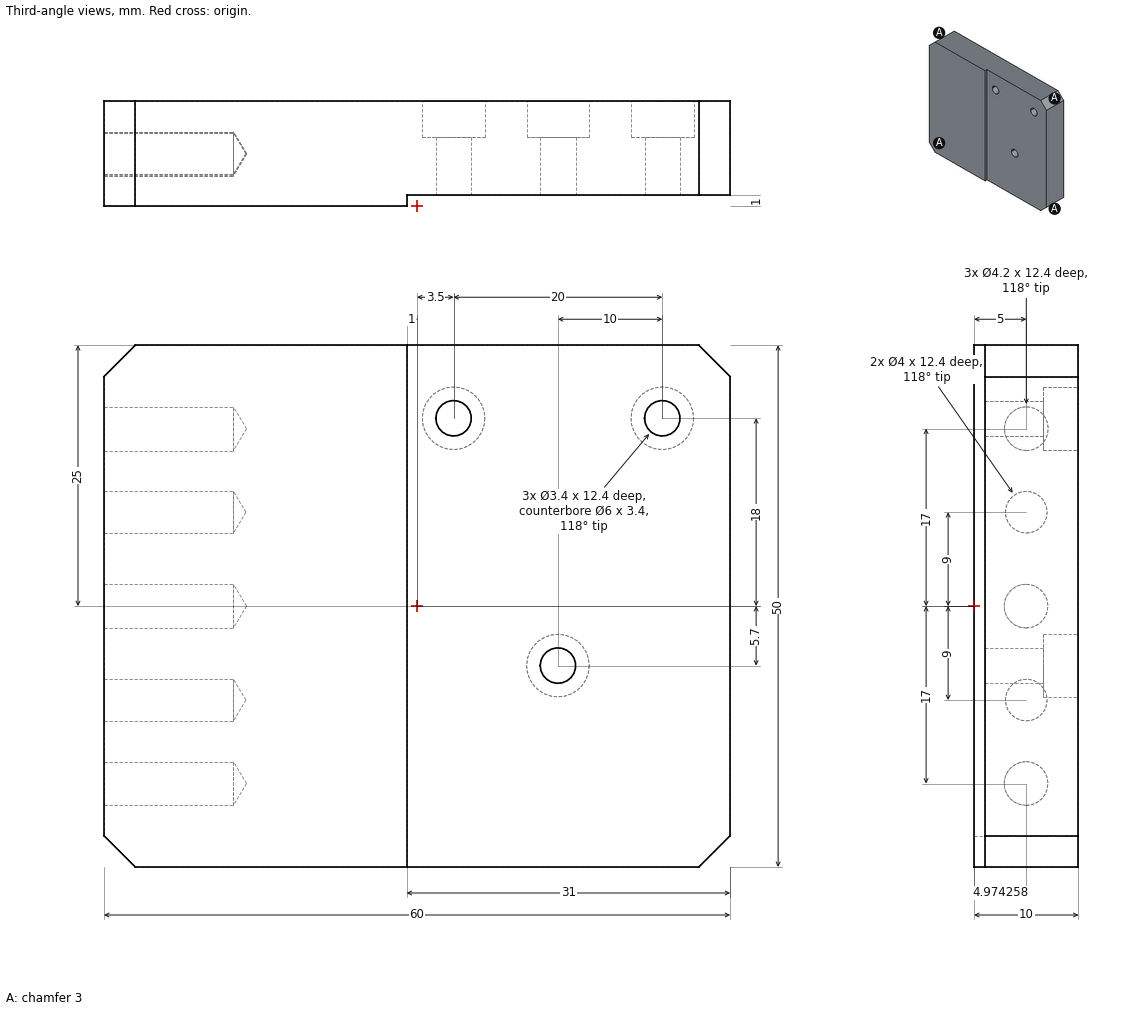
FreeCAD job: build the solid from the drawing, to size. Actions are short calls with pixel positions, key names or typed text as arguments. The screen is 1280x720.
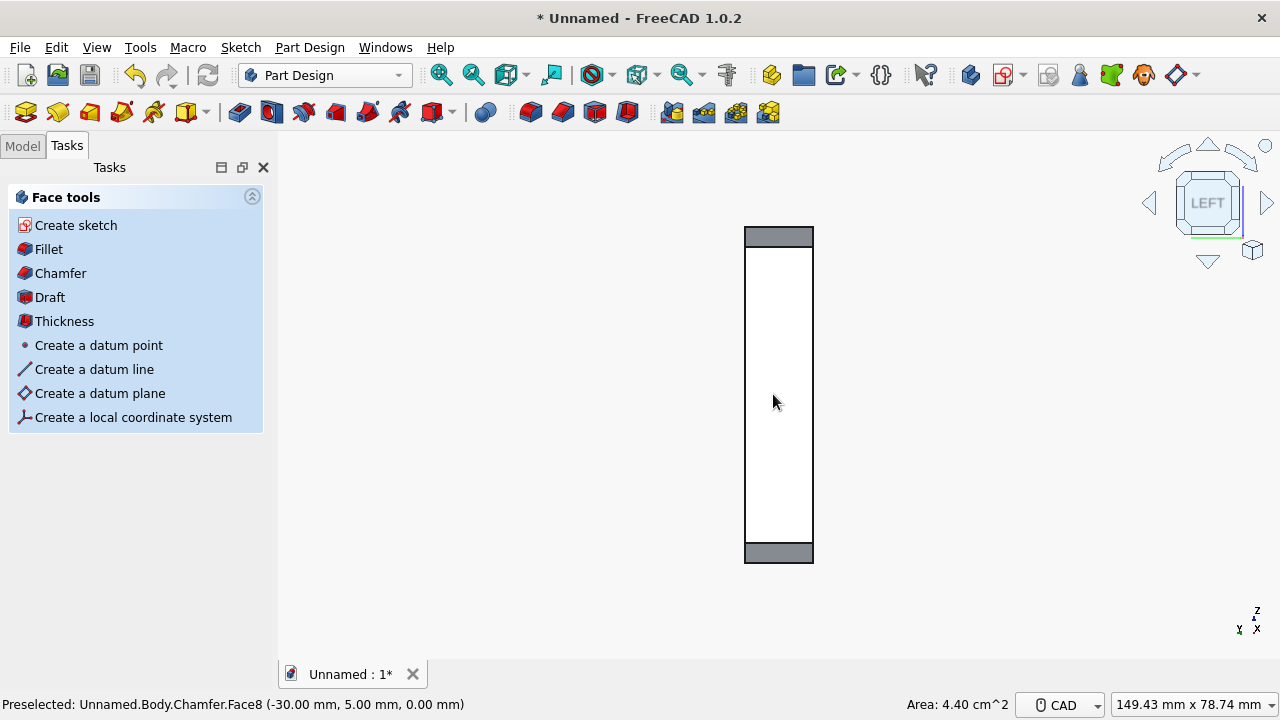
click(1004, 76)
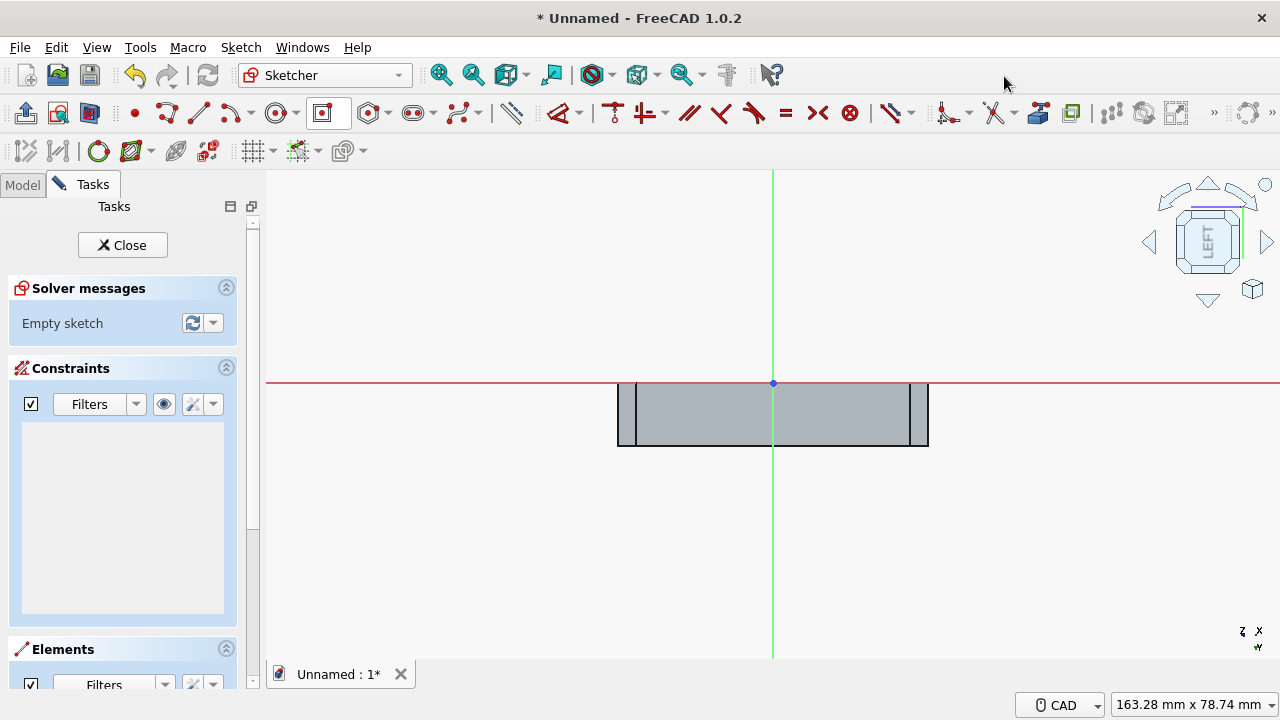
scroll(829, 398, up, 4)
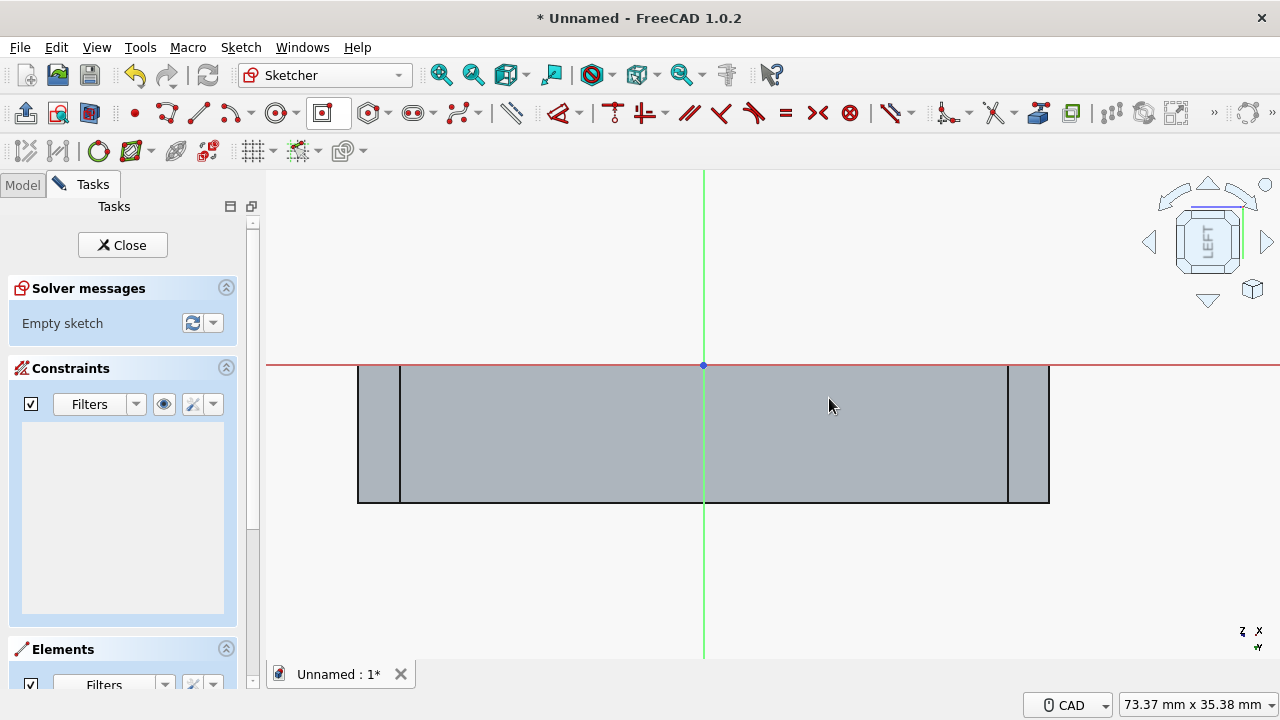
click(276, 114)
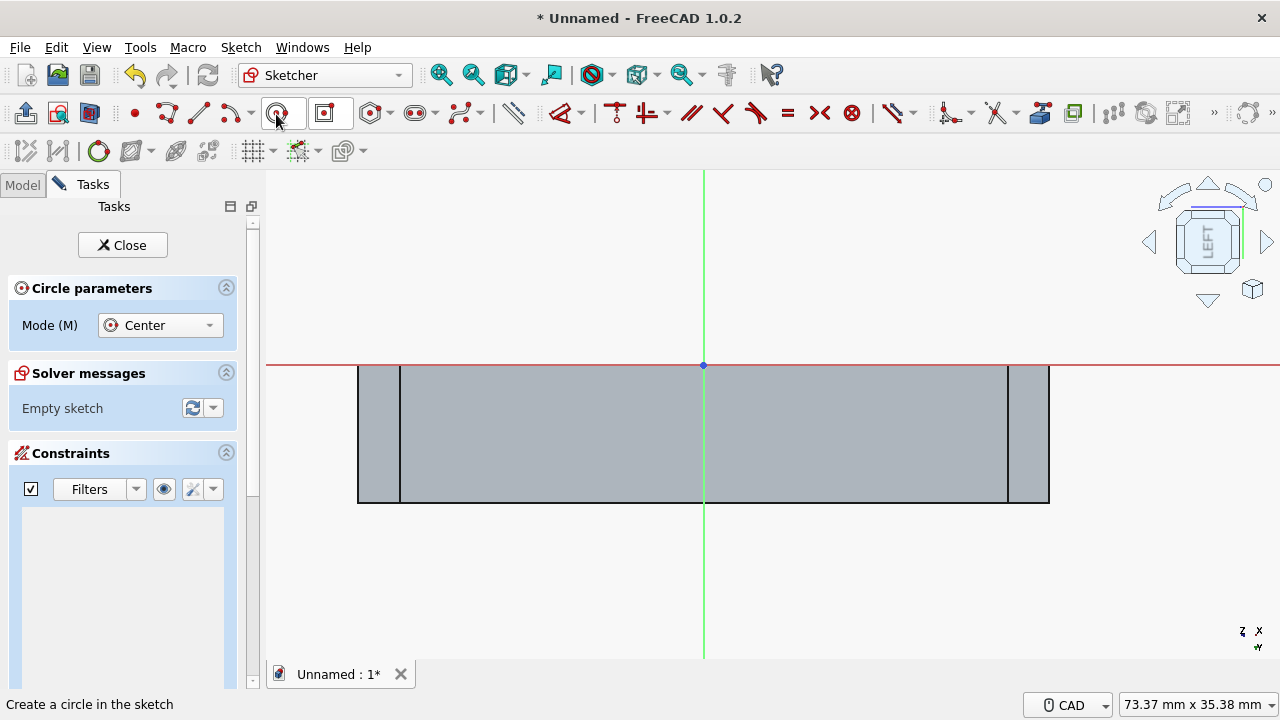
click(469, 434)
move(489, 414)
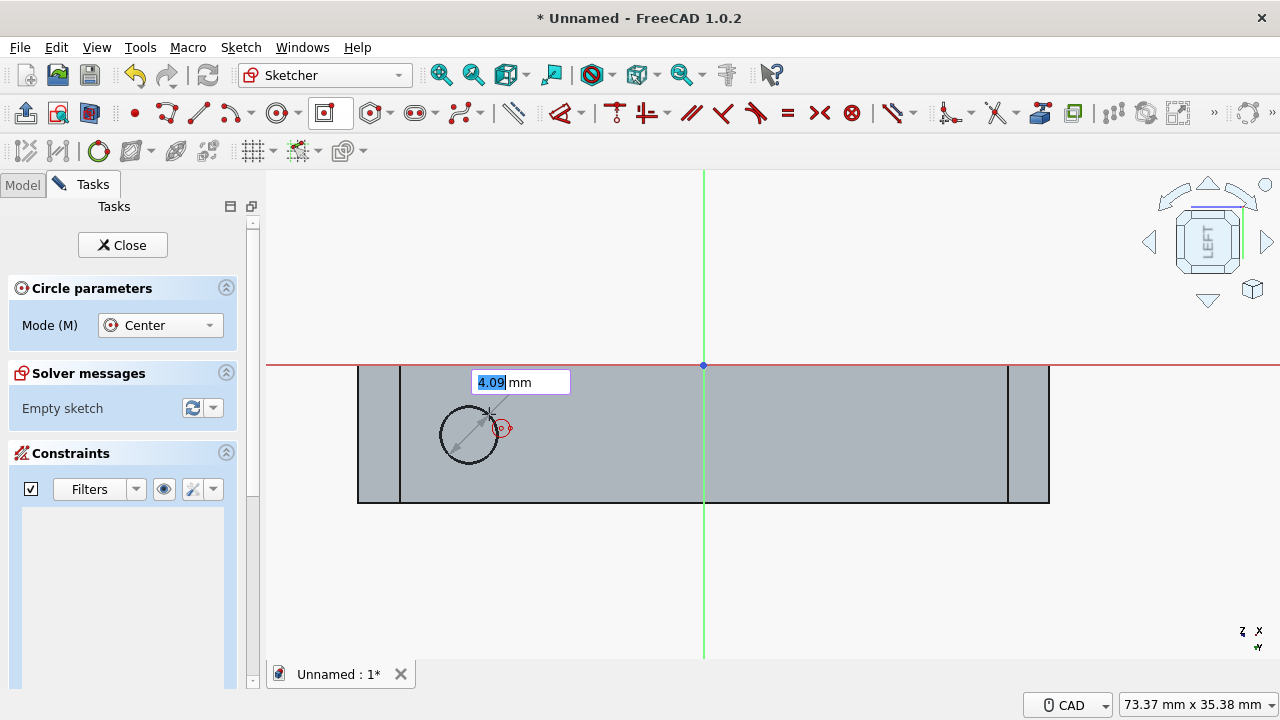
text(4.2)
key(Return)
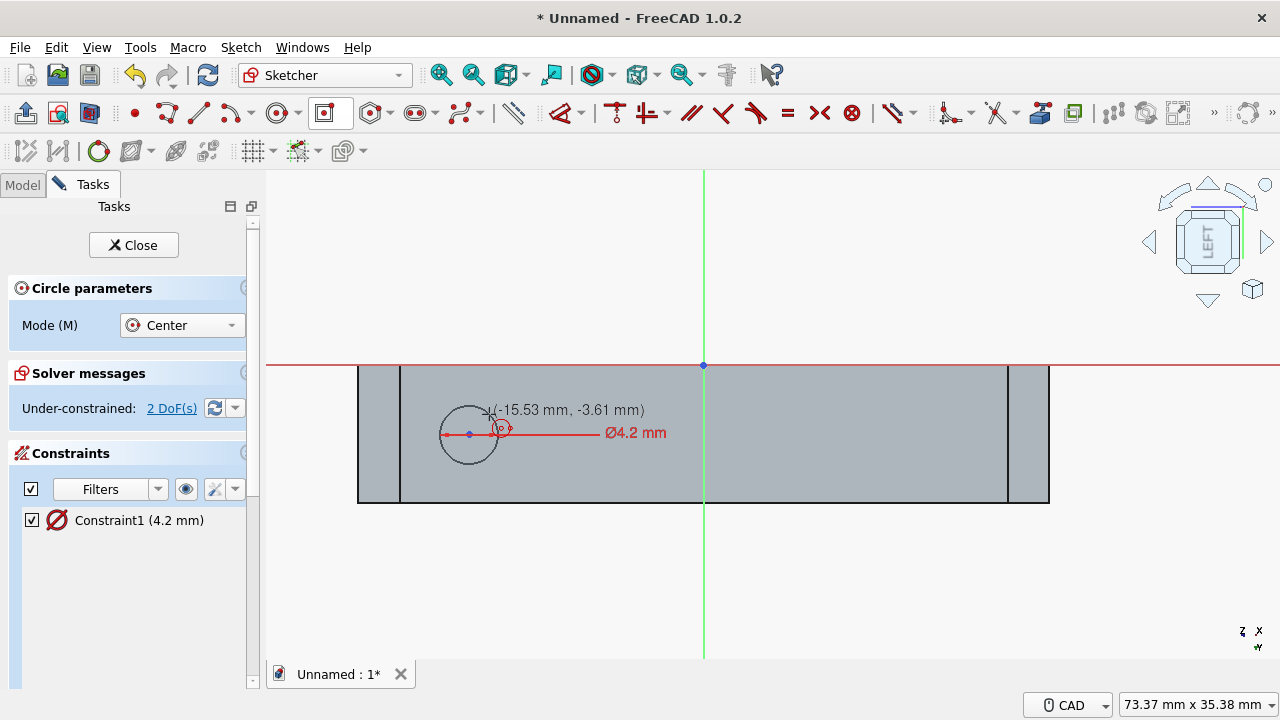
click(939, 434)
move(959, 413)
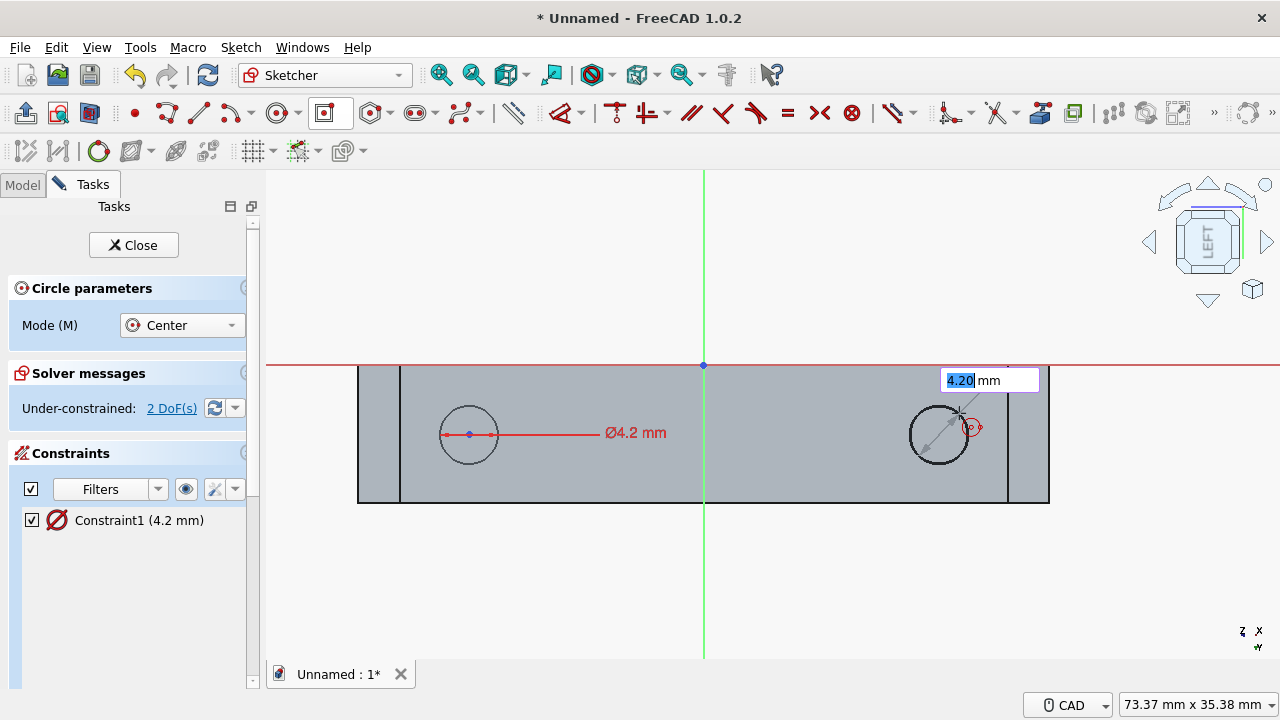
text(4.2)
key(Return)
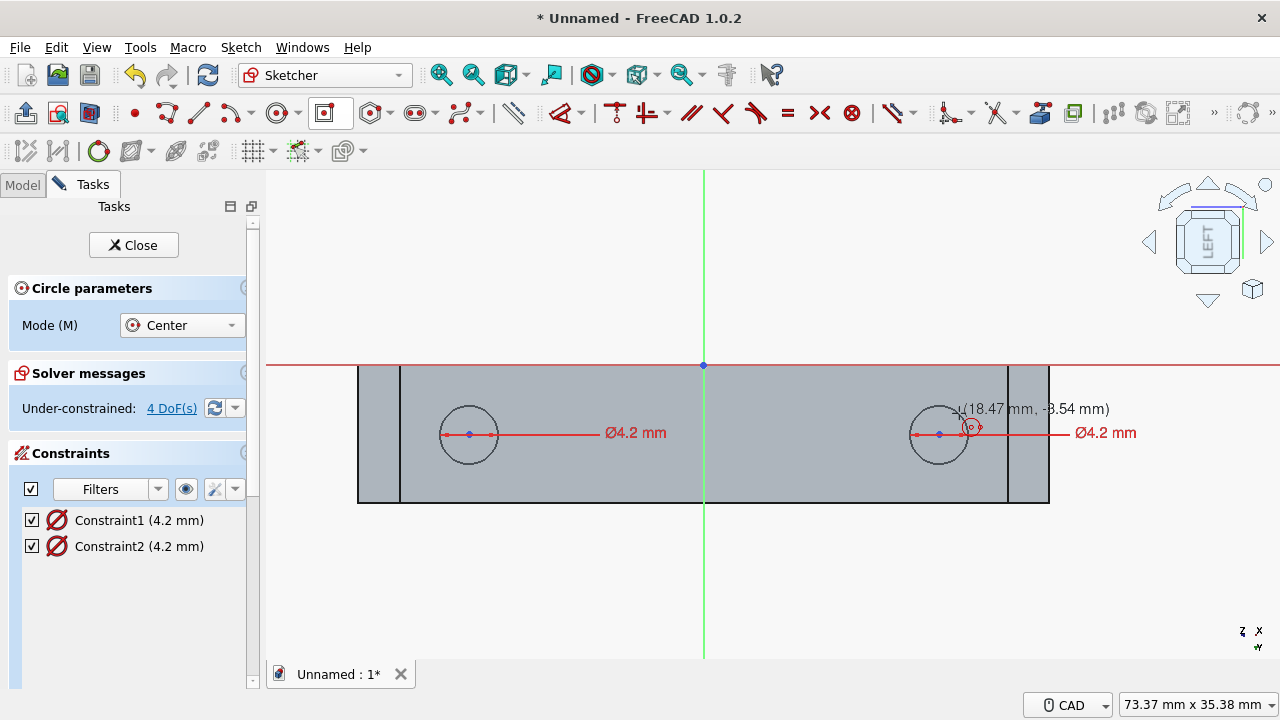
click(704, 434)
move(724, 413)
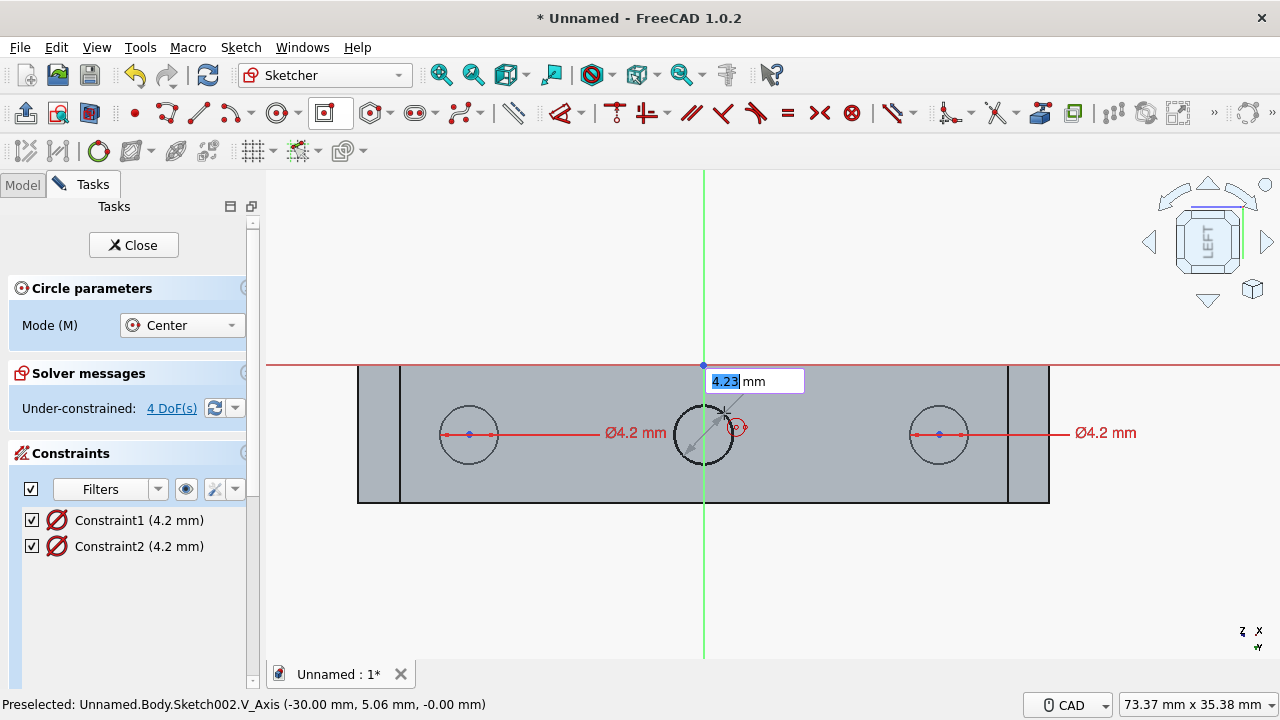
text(4.2)
key(Return)
key(Escape)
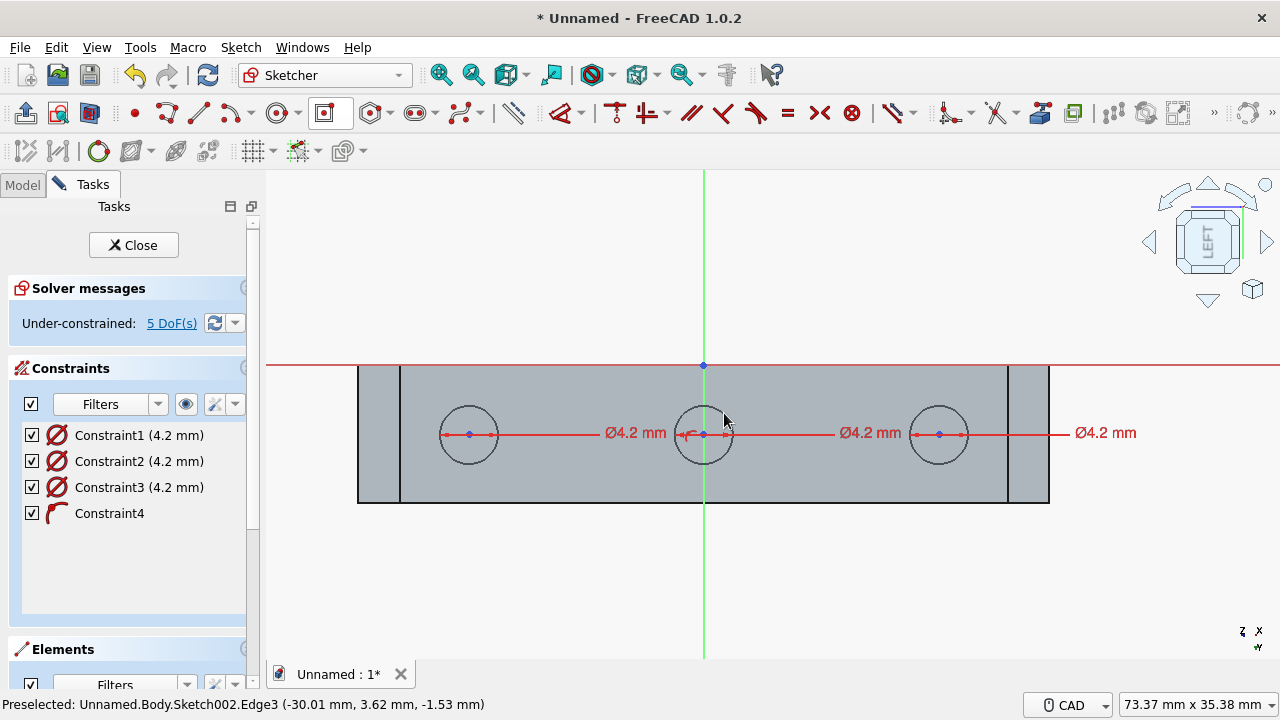
click(939, 435)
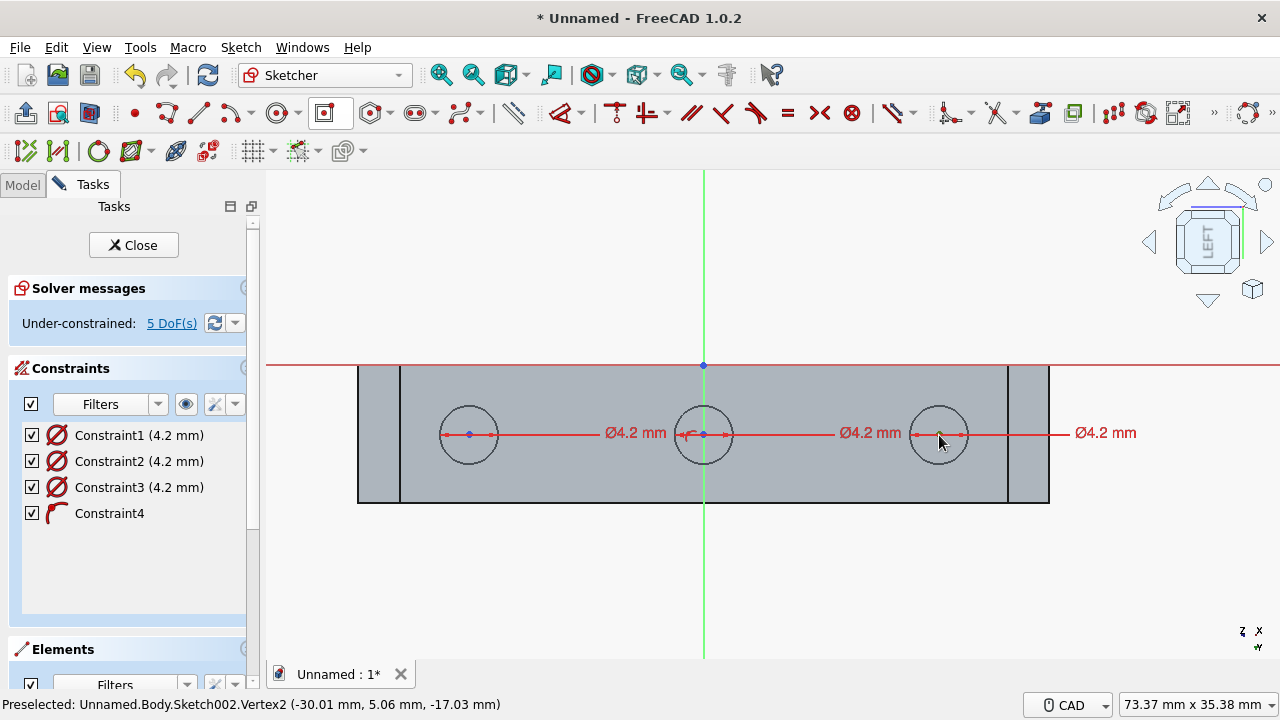
click(704, 435)